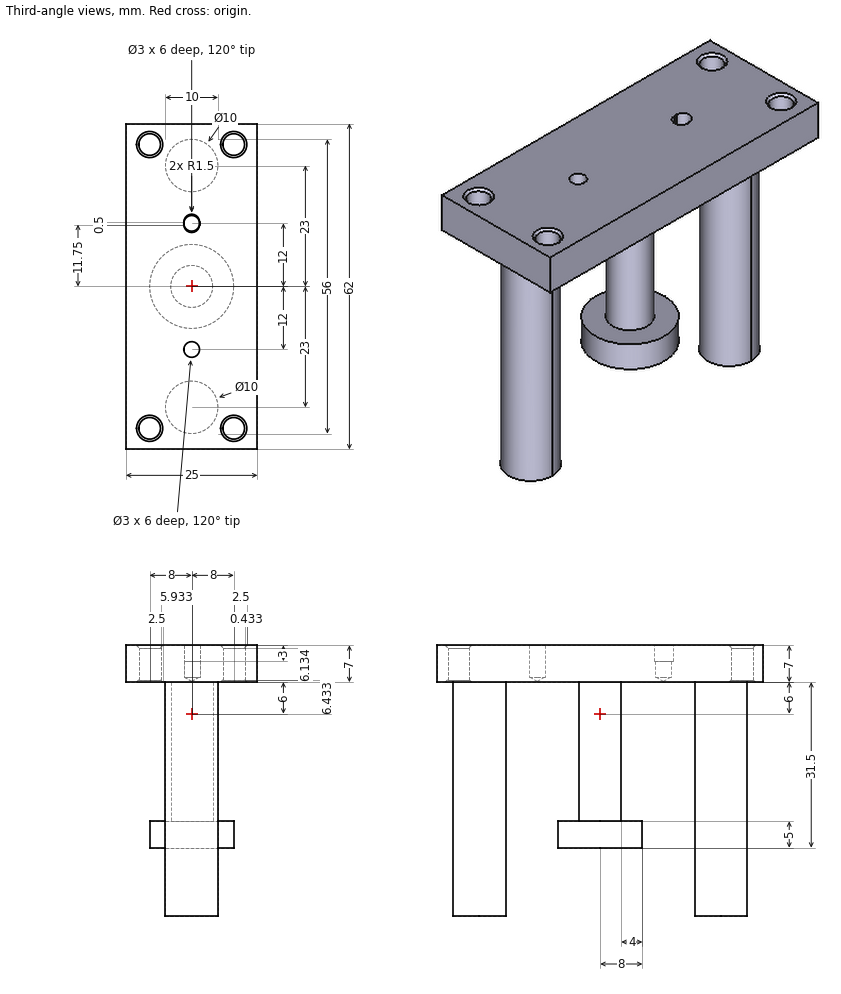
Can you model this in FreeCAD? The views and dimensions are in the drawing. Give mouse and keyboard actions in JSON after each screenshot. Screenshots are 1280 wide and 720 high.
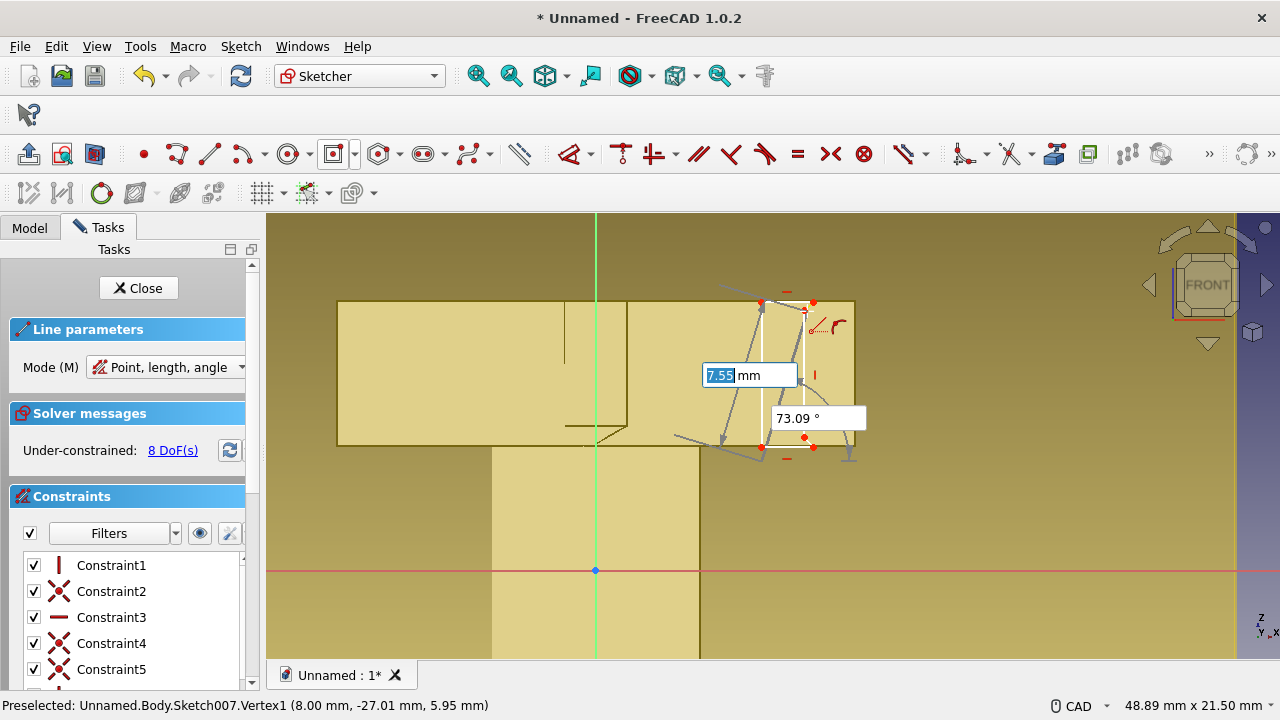
{"action": "left_click", "coordinate": [762, 505]}
{"action": "key", "text": "Escape"}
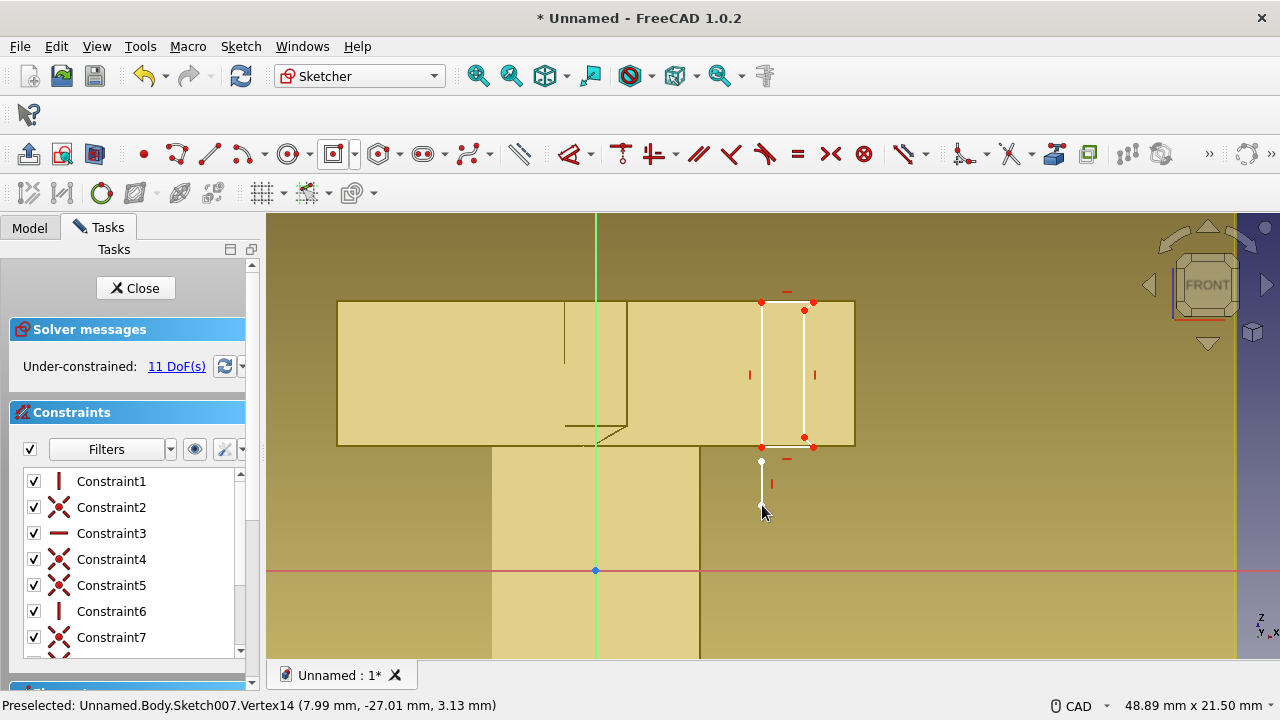
{"action": "left_click", "coordinate": [762, 475]}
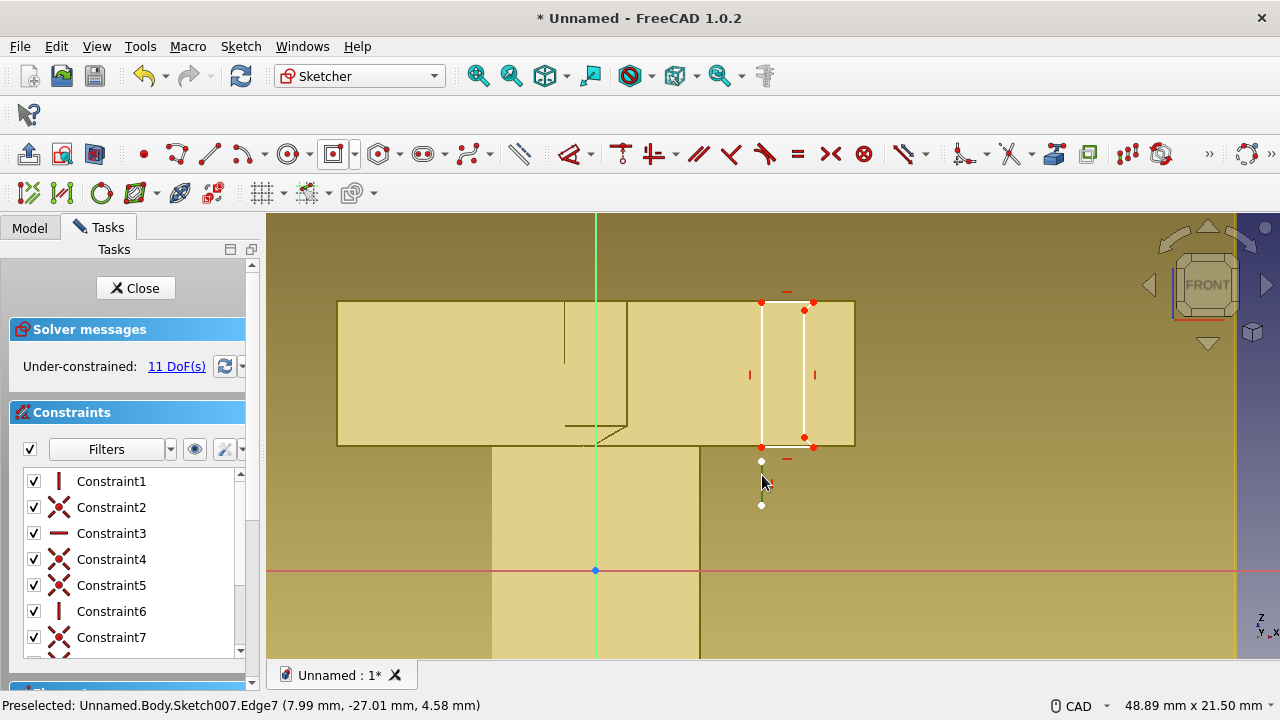
{"action": "left_click", "coordinate": [520, 154]}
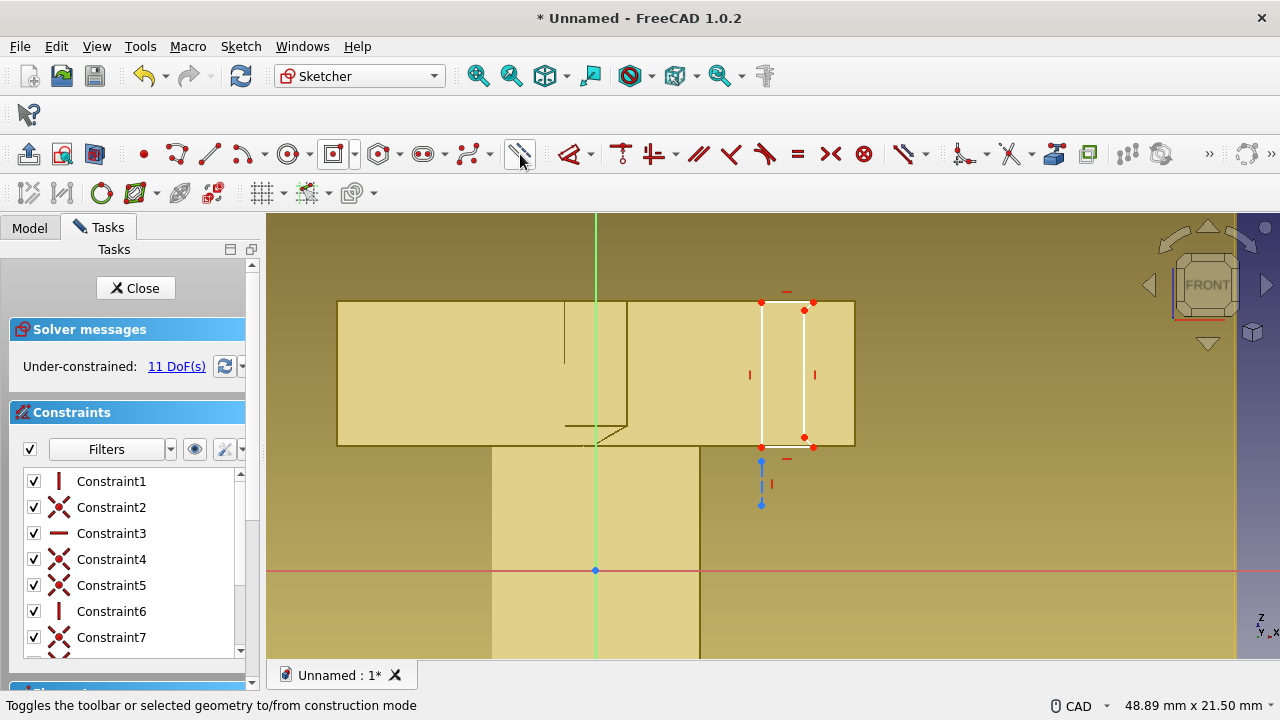
{"action": "left_click", "coordinate": [568, 154]}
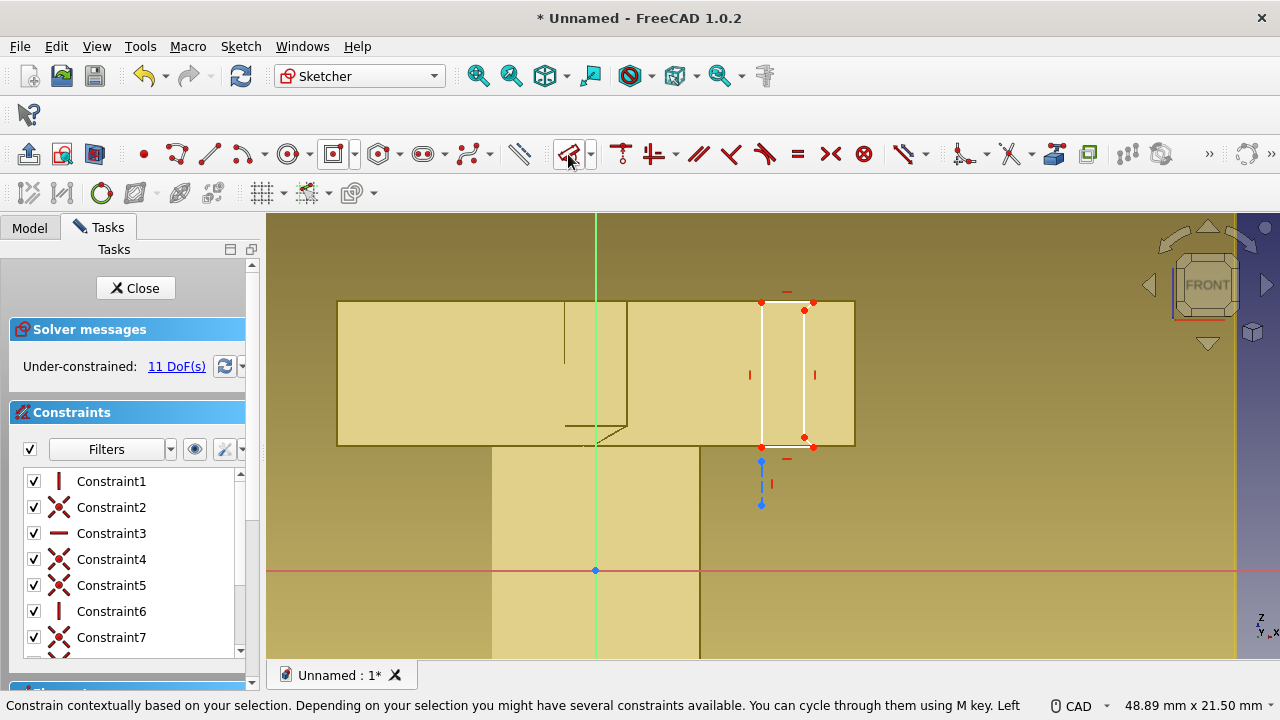
{"action": "left_click", "coordinate": [762, 404]}
{"action": "left_click", "coordinate": [728, 375]}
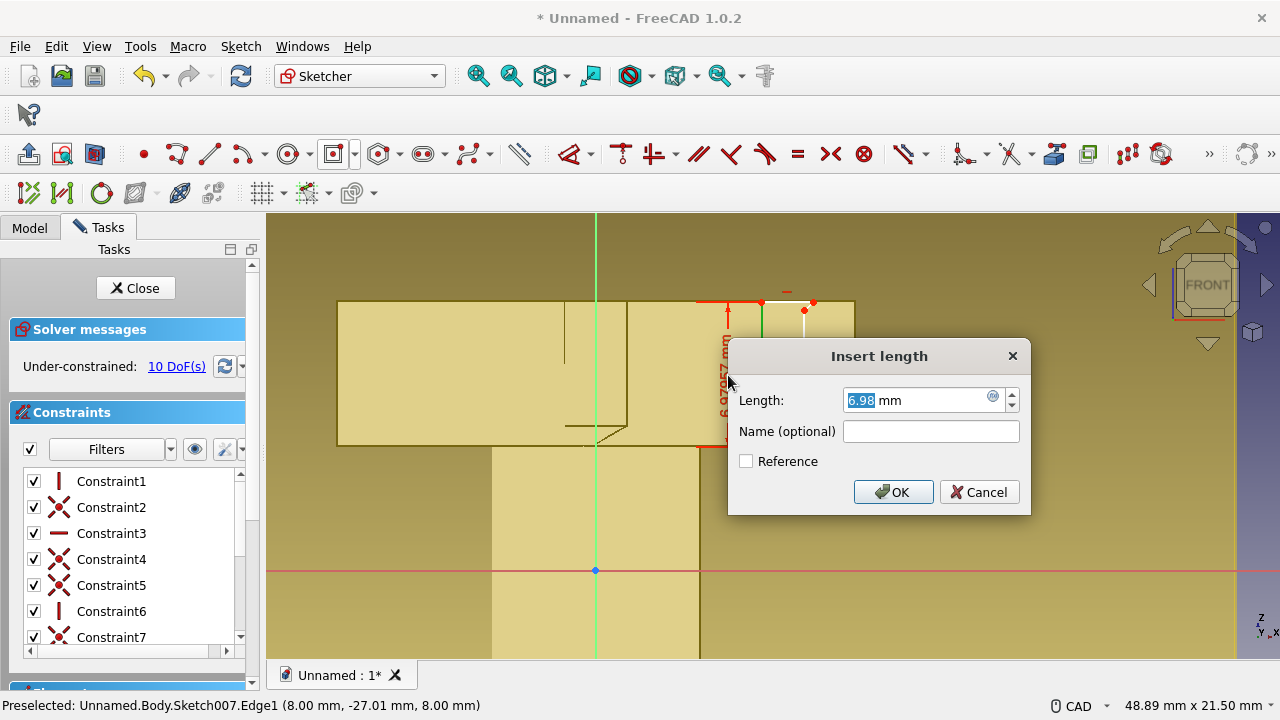
{"action": "type", "text": "7"}
{"action": "key", "text": "Return"}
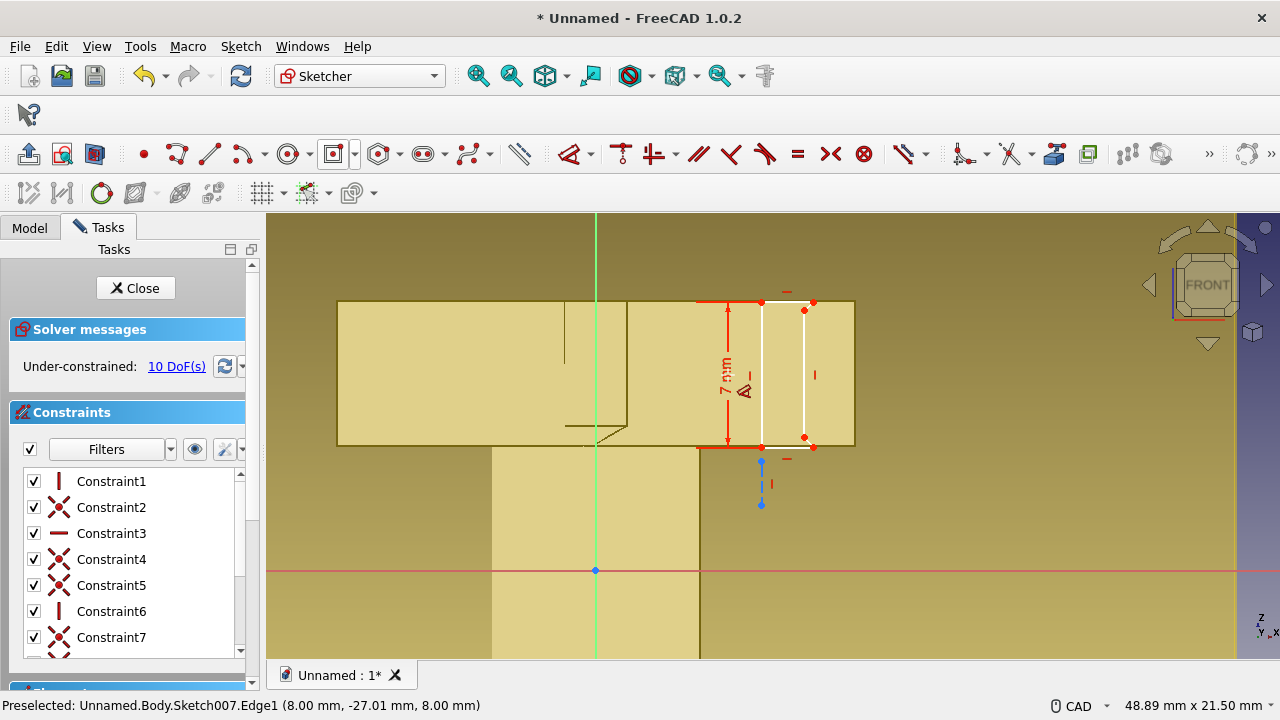
{"action": "left_click", "coordinate": [762, 448]}
{"action": "left_click", "coordinate": [679, 605]}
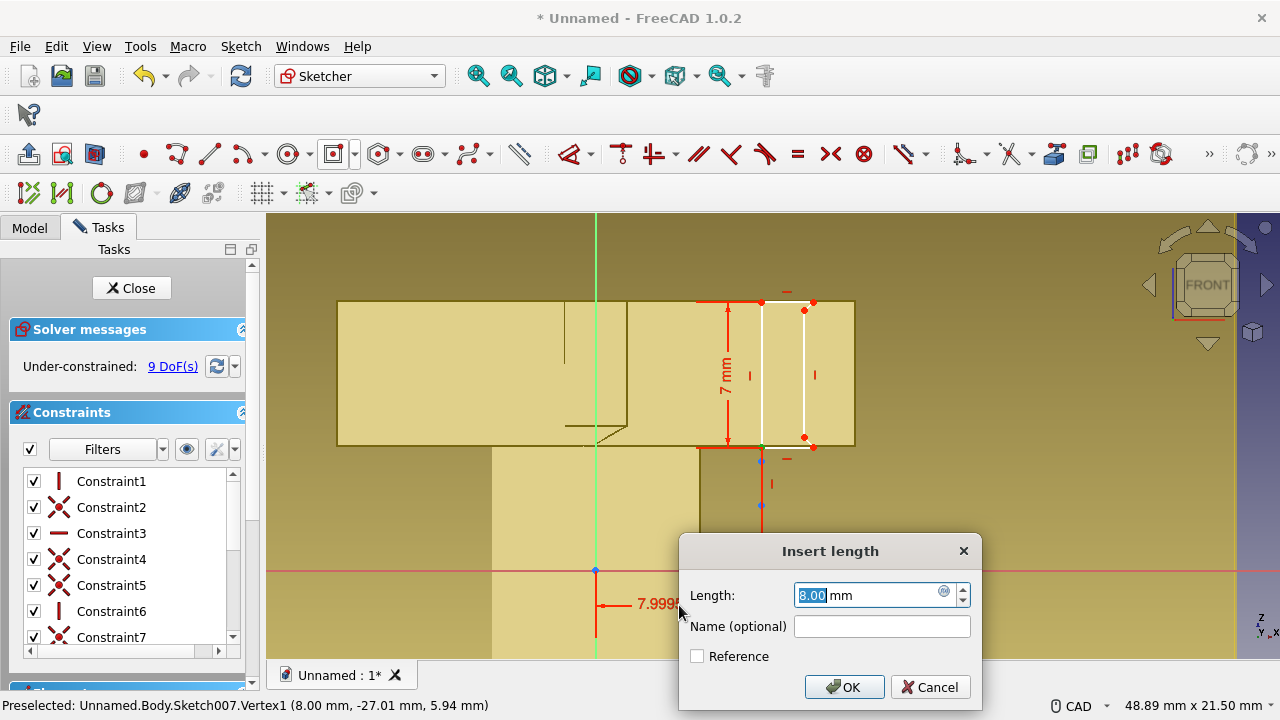
{"action": "type", "text": "8"}
{"action": "key", "text": "Return"}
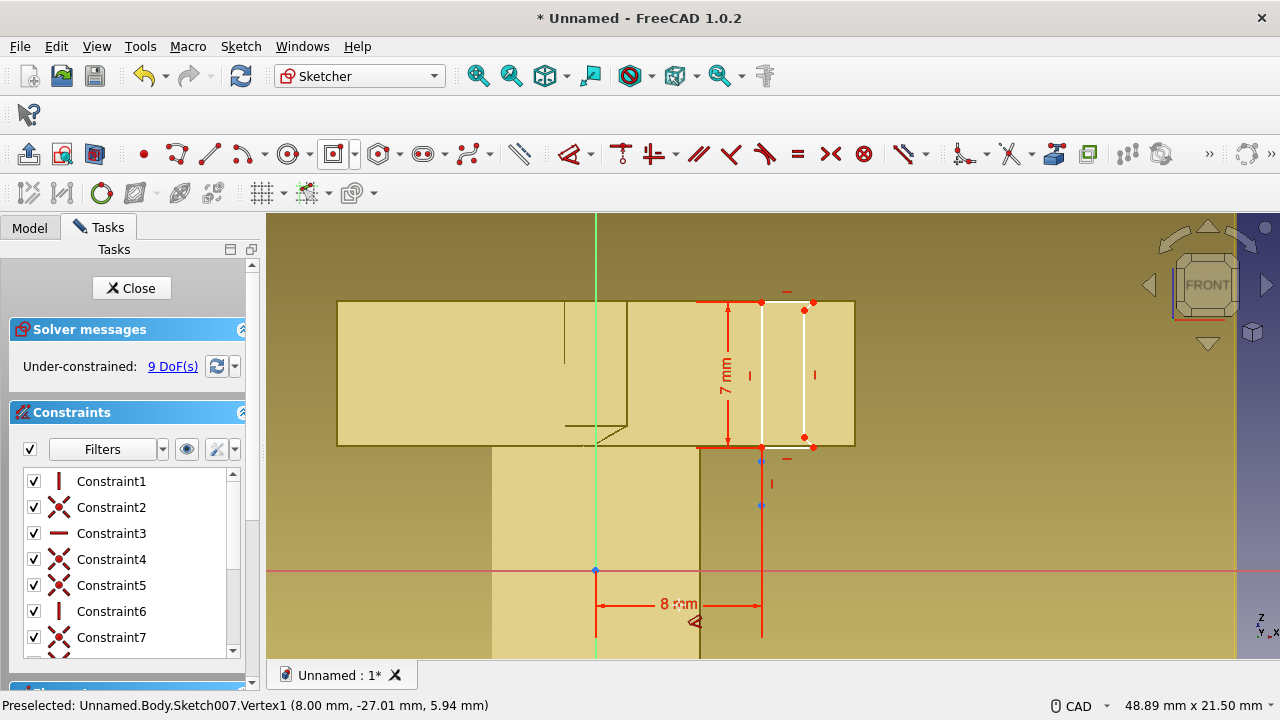
{"action": "left_click", "coordinate": [762, 448]}
{"action": "left_click", "coordinate": [562, 509]}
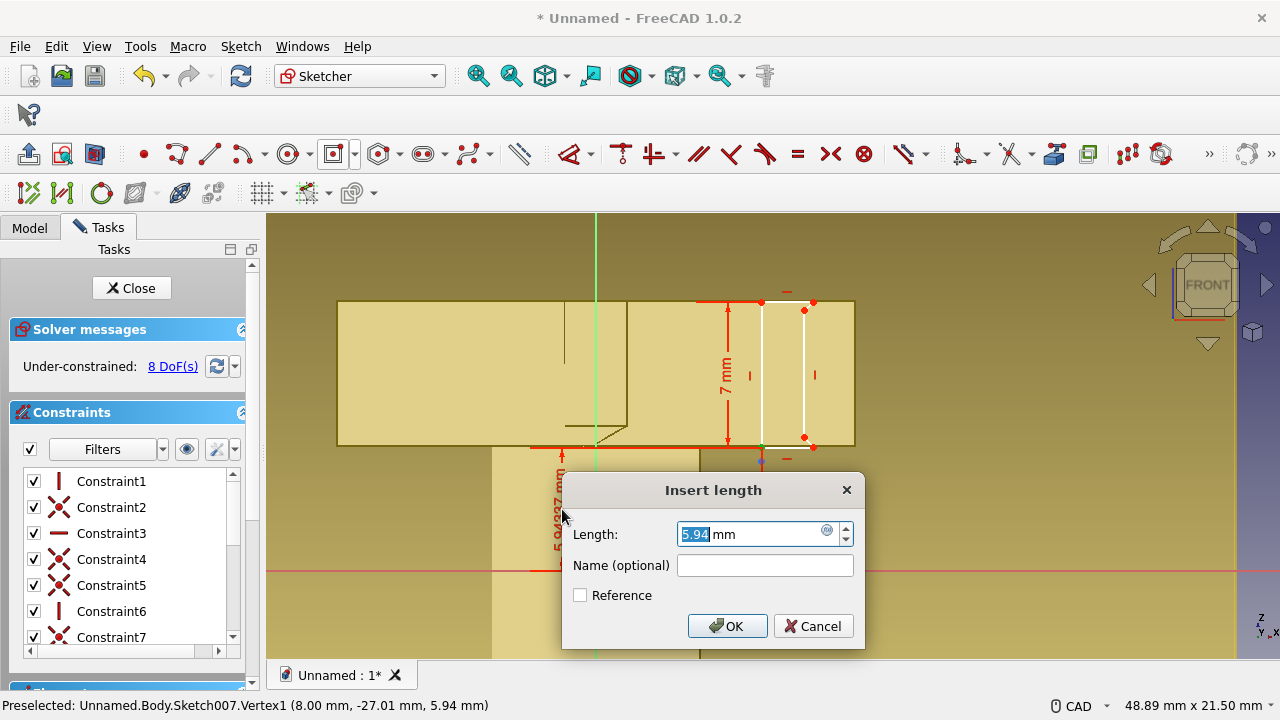
{"action": "type", "text": "6"}
{"action": "key", "text": "Return"}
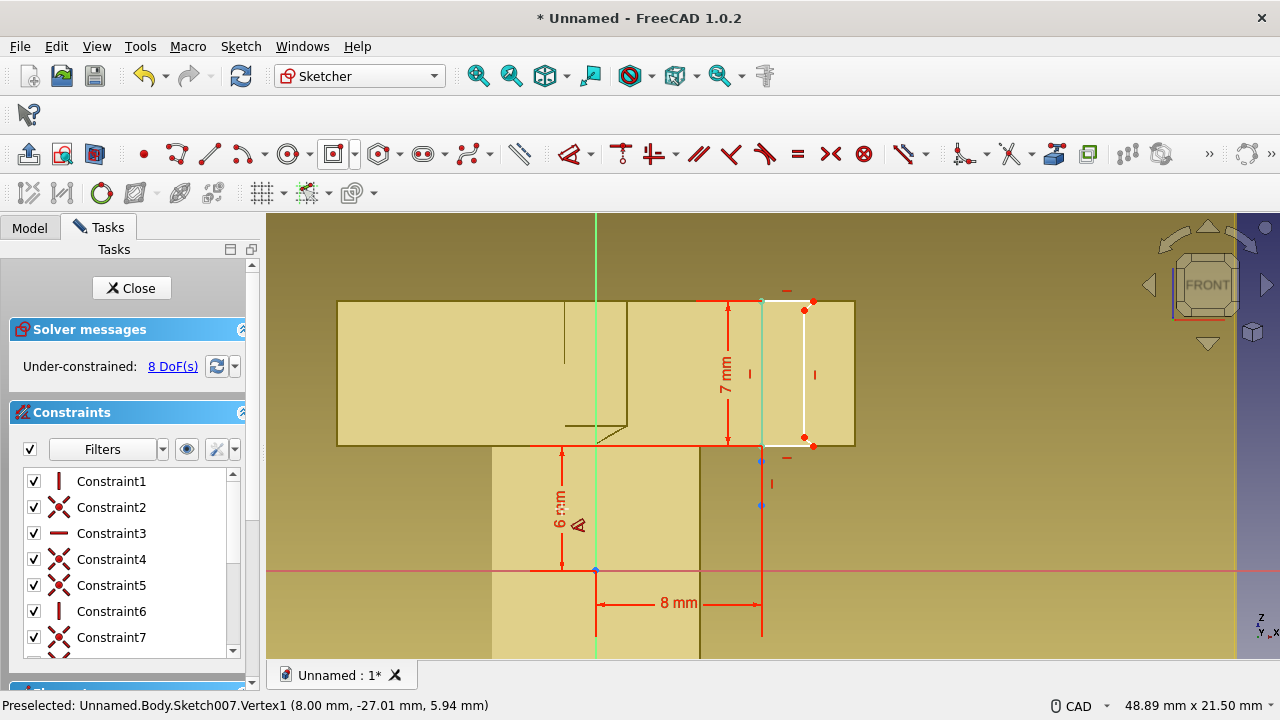
{"action": "left_click", "coordinate": [762, 461]}
{"action": "left_click", "coordinate": [679, 427]}